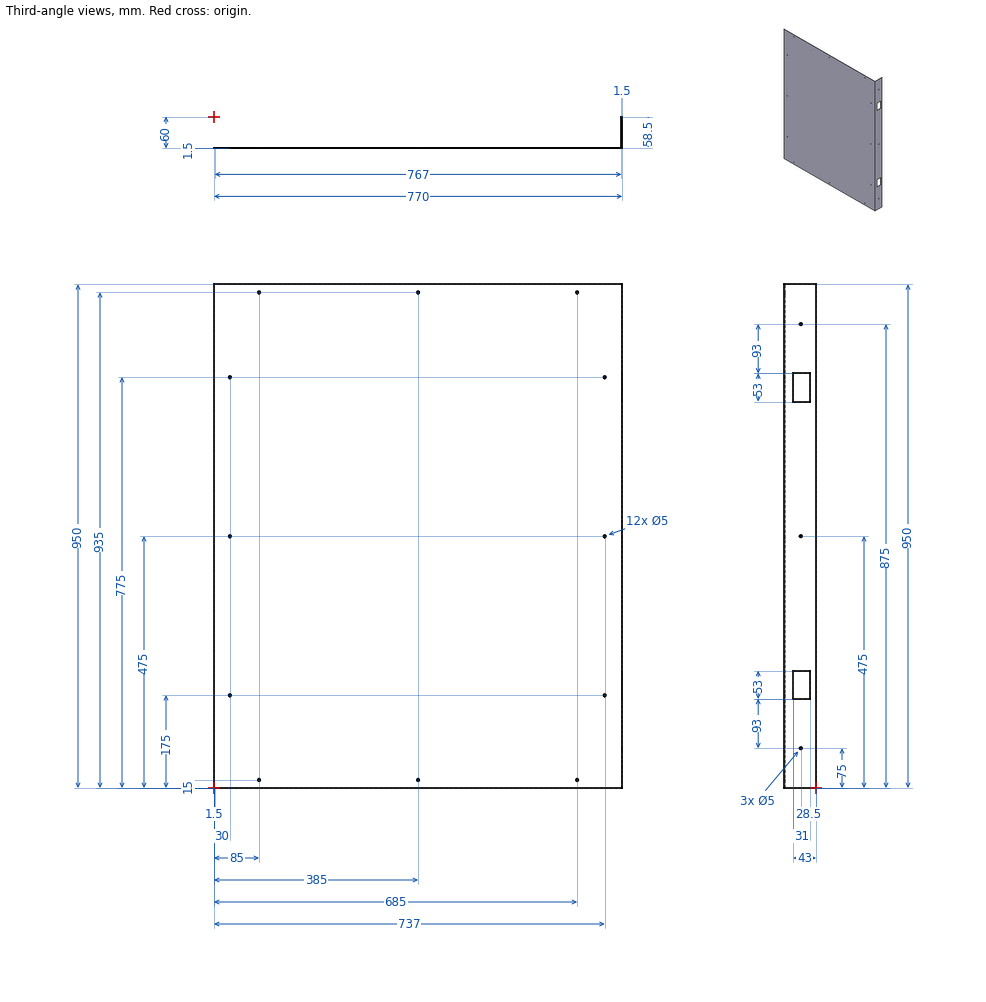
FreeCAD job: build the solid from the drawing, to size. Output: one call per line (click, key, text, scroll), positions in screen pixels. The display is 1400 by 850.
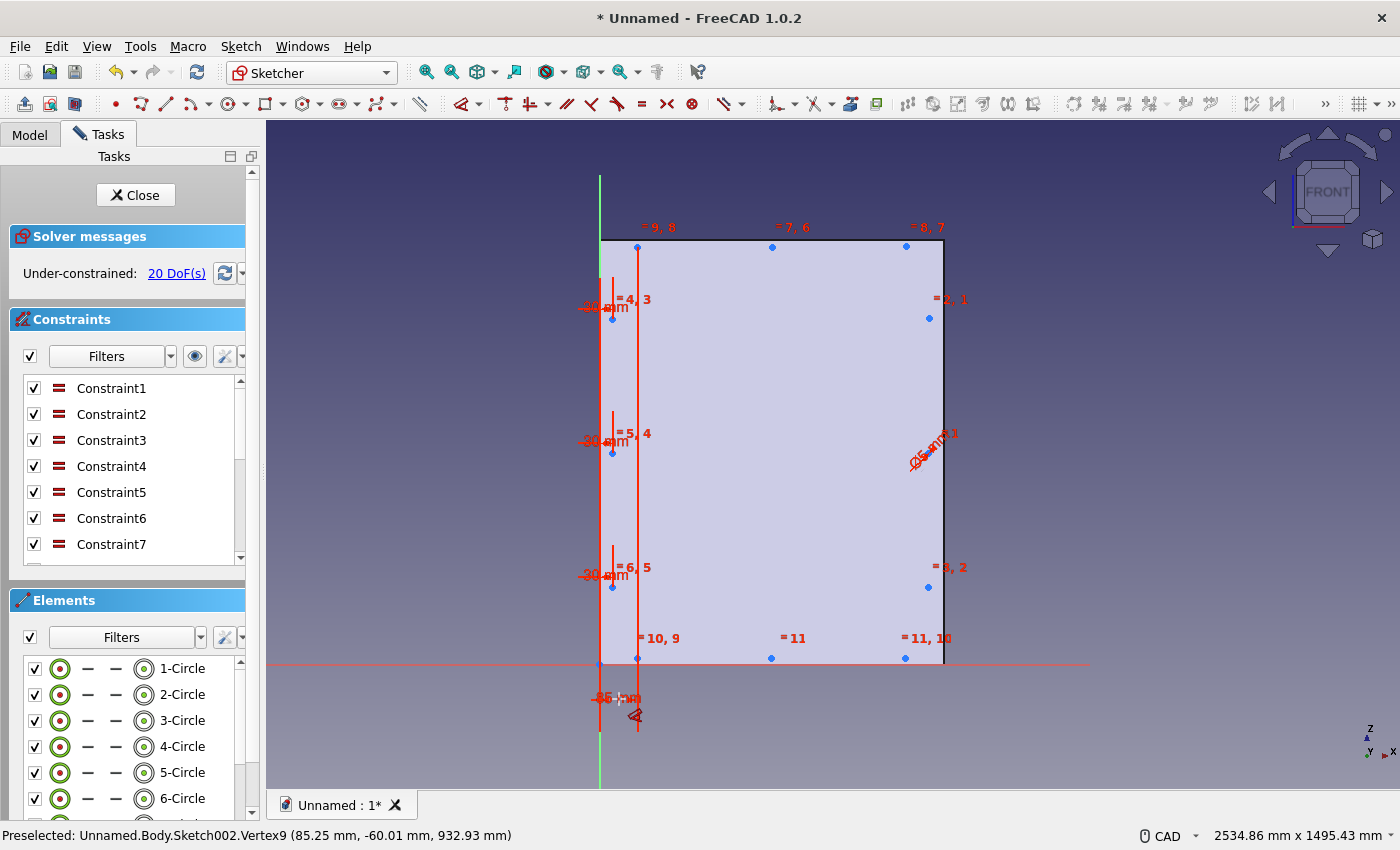
click(638, 658)
click(619, 624)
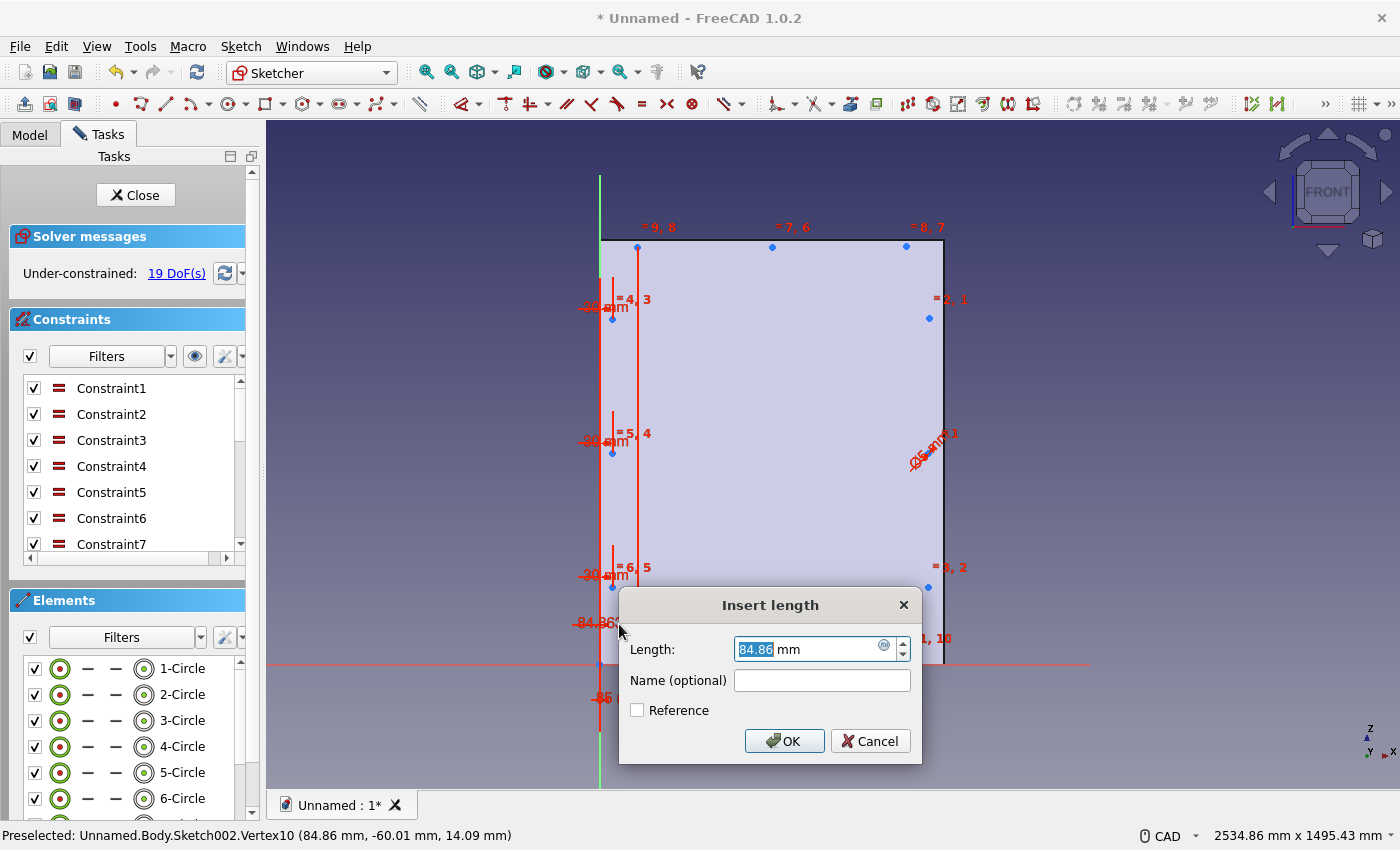
text(85)
key(Return)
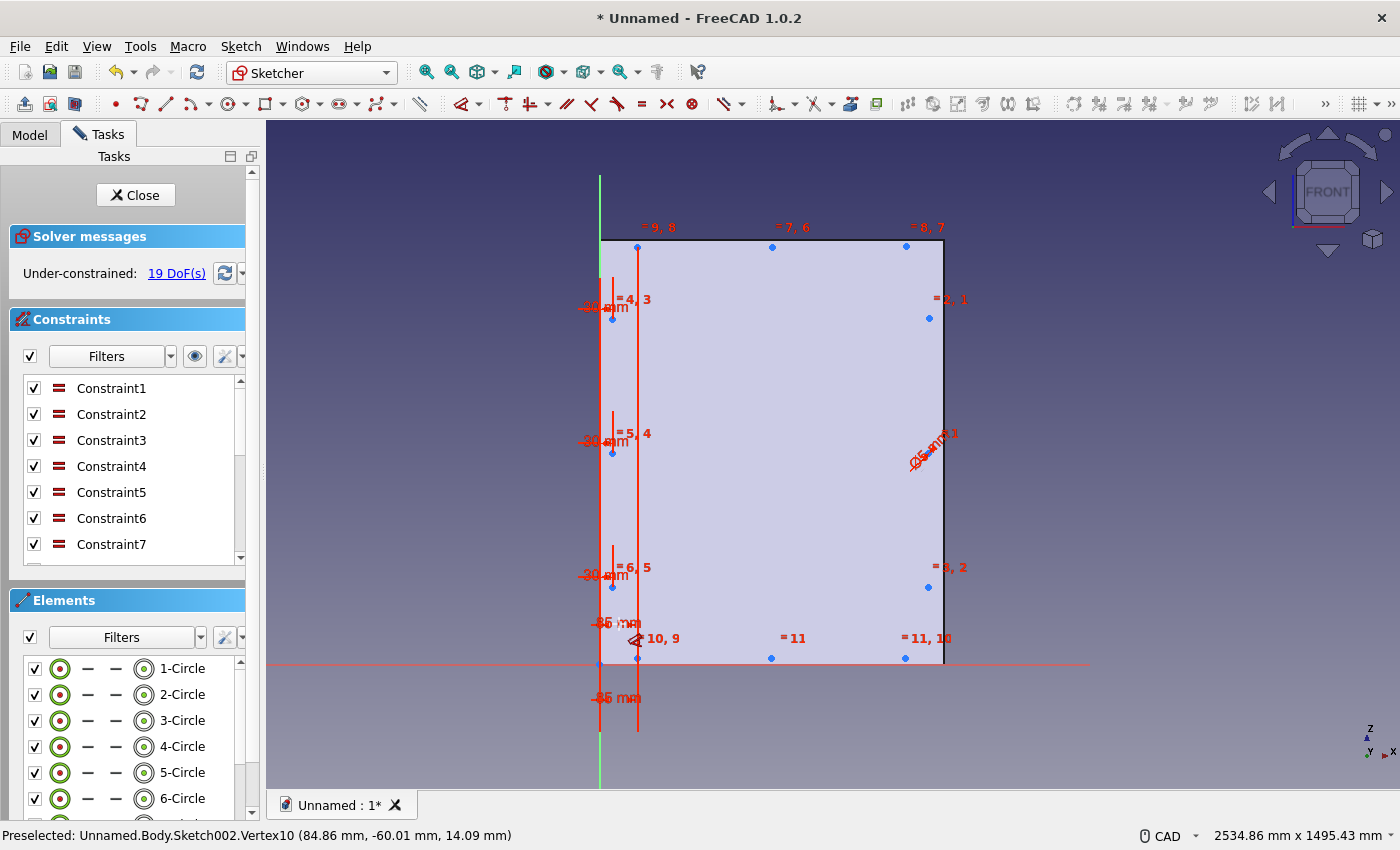
scroll(638, 658, up, 9)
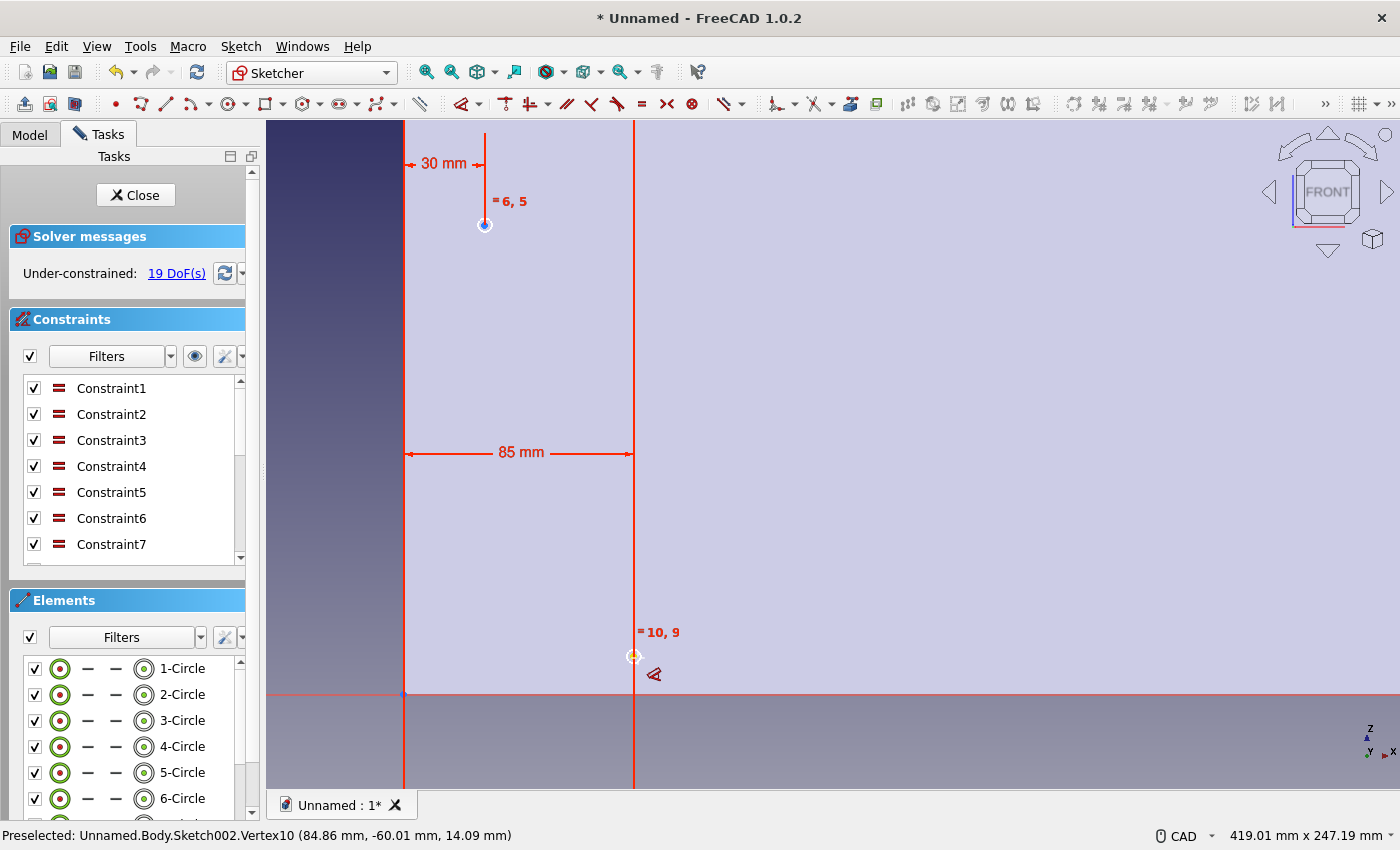
click(634, 657)
click(370, 676)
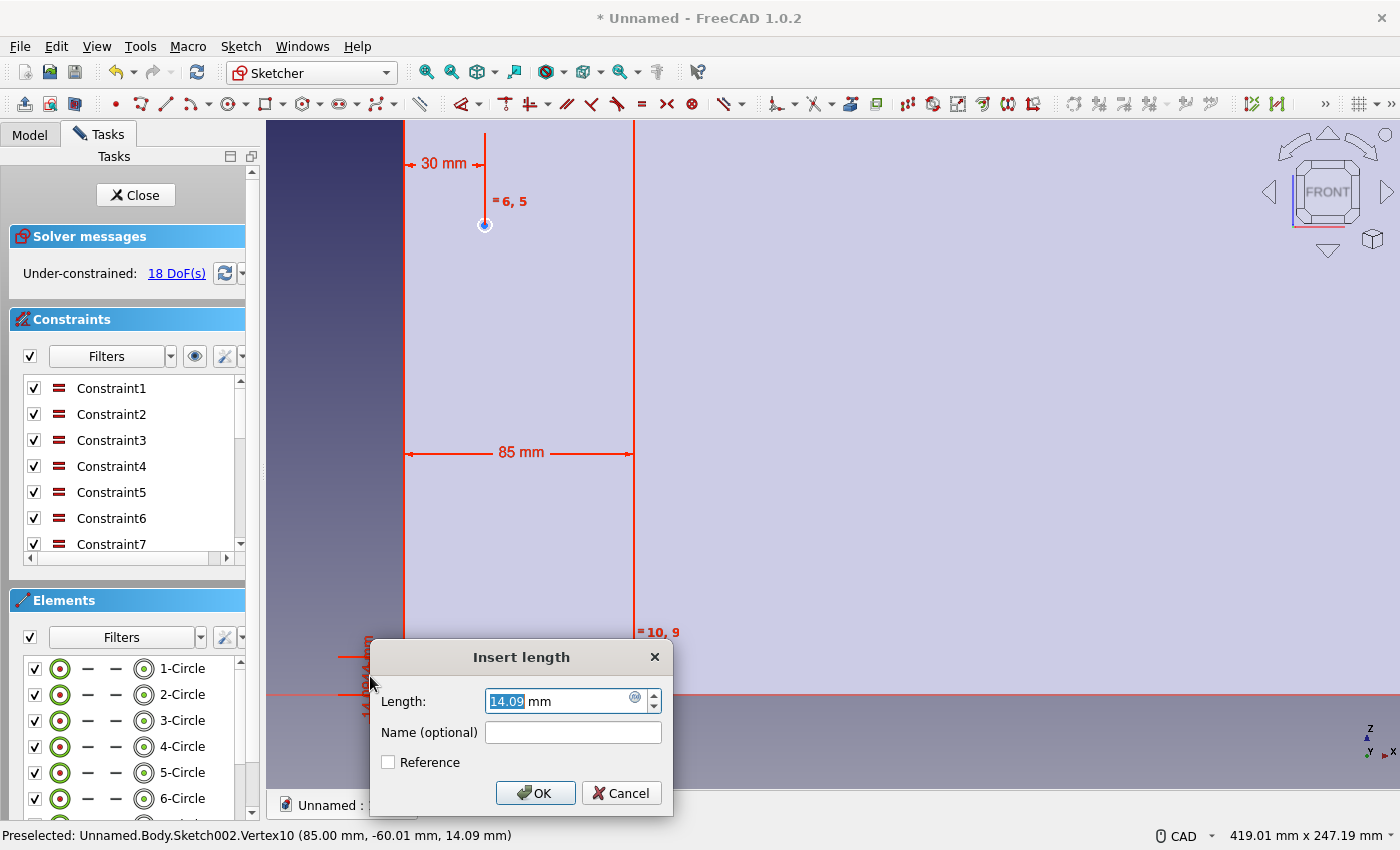
text(15)
key(Return)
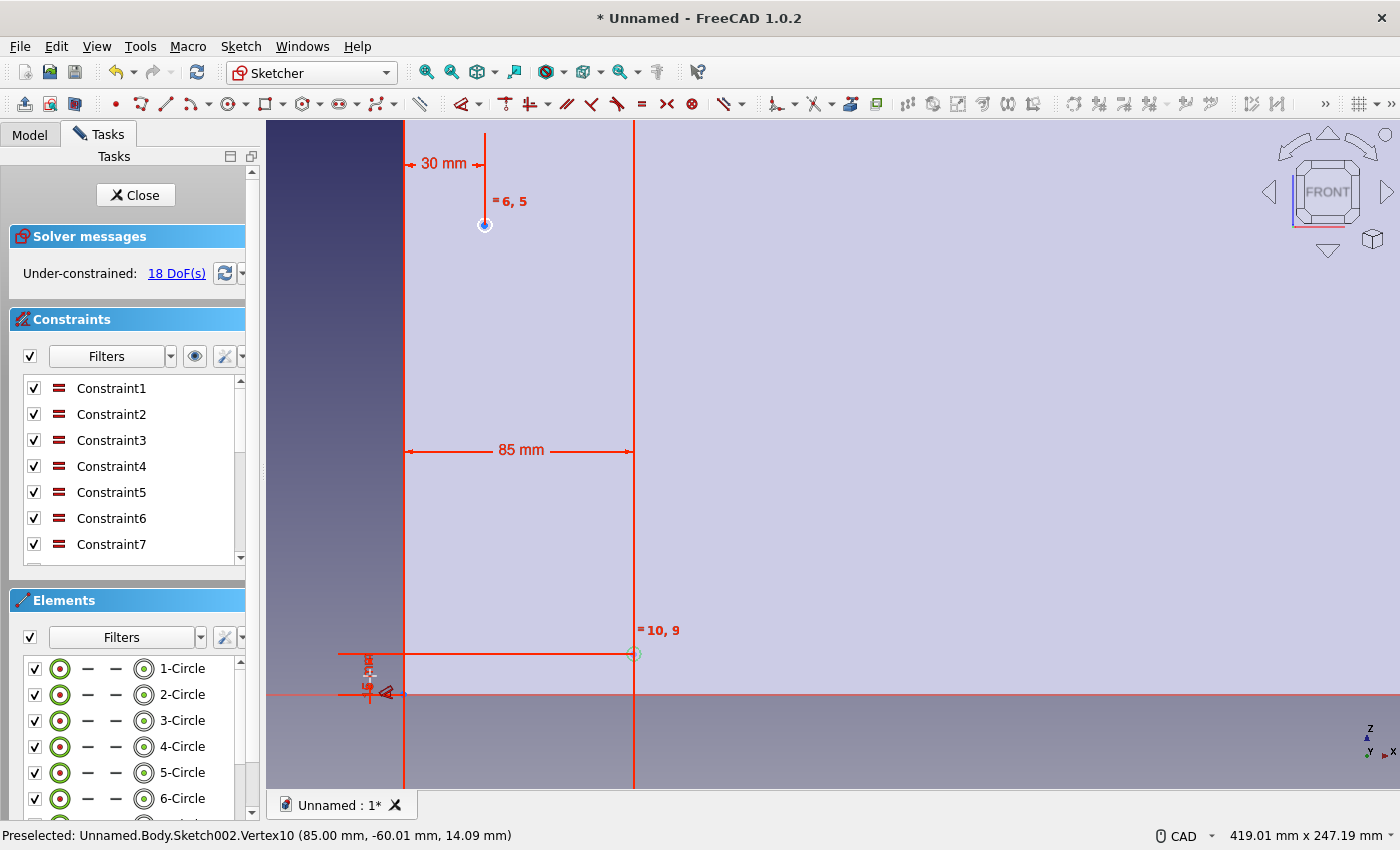
scroll(638, 658, down, 9)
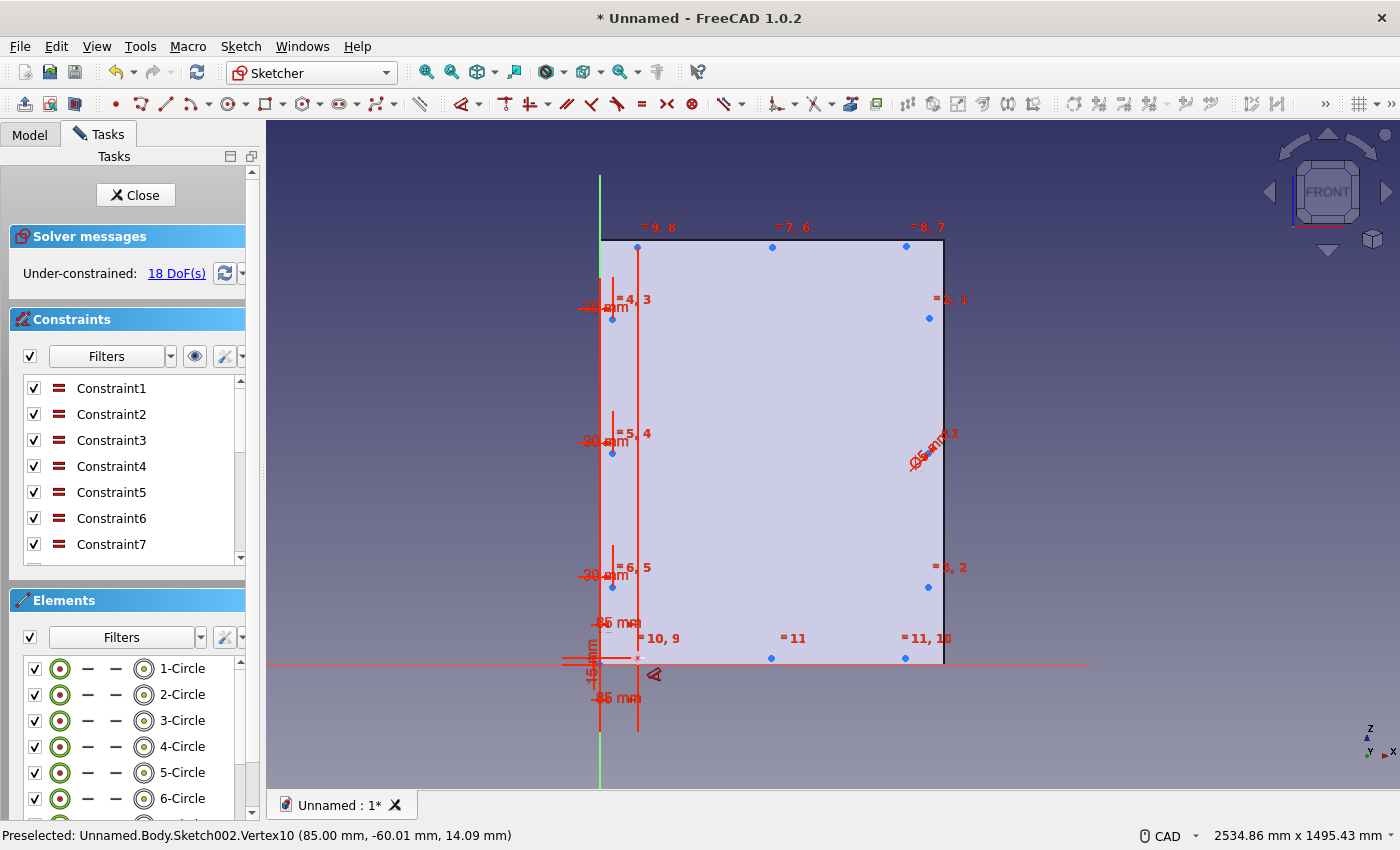
scroll(906, 658, up, 9)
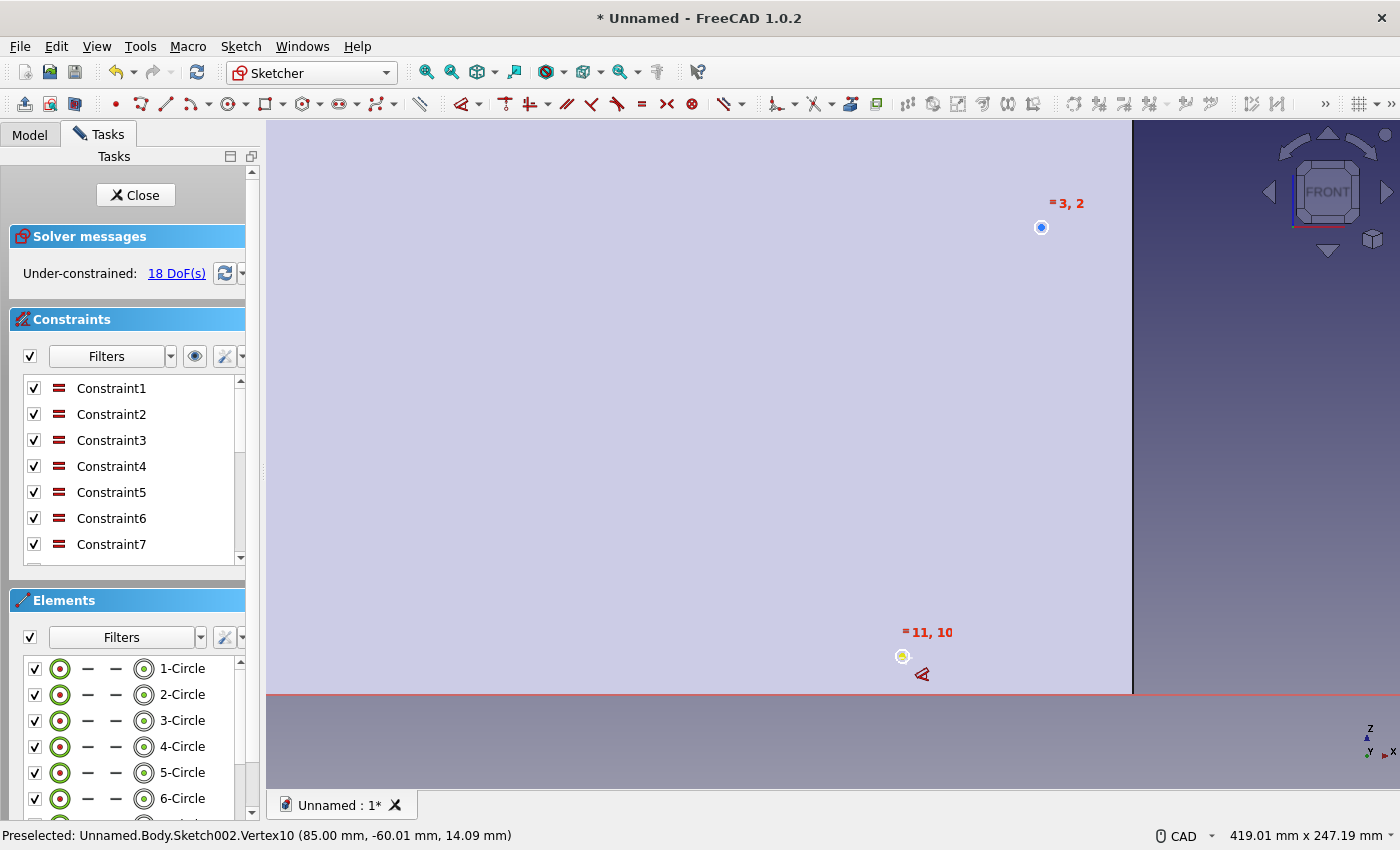
click(903, 656)
click(937, 675)